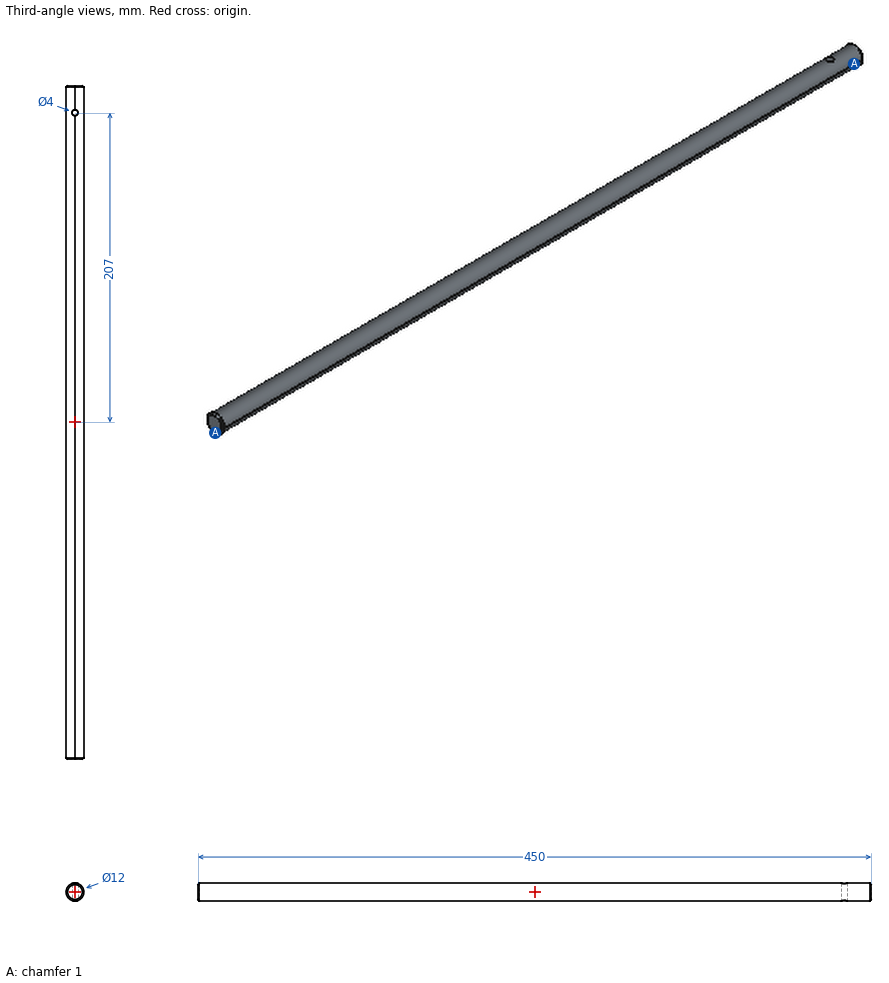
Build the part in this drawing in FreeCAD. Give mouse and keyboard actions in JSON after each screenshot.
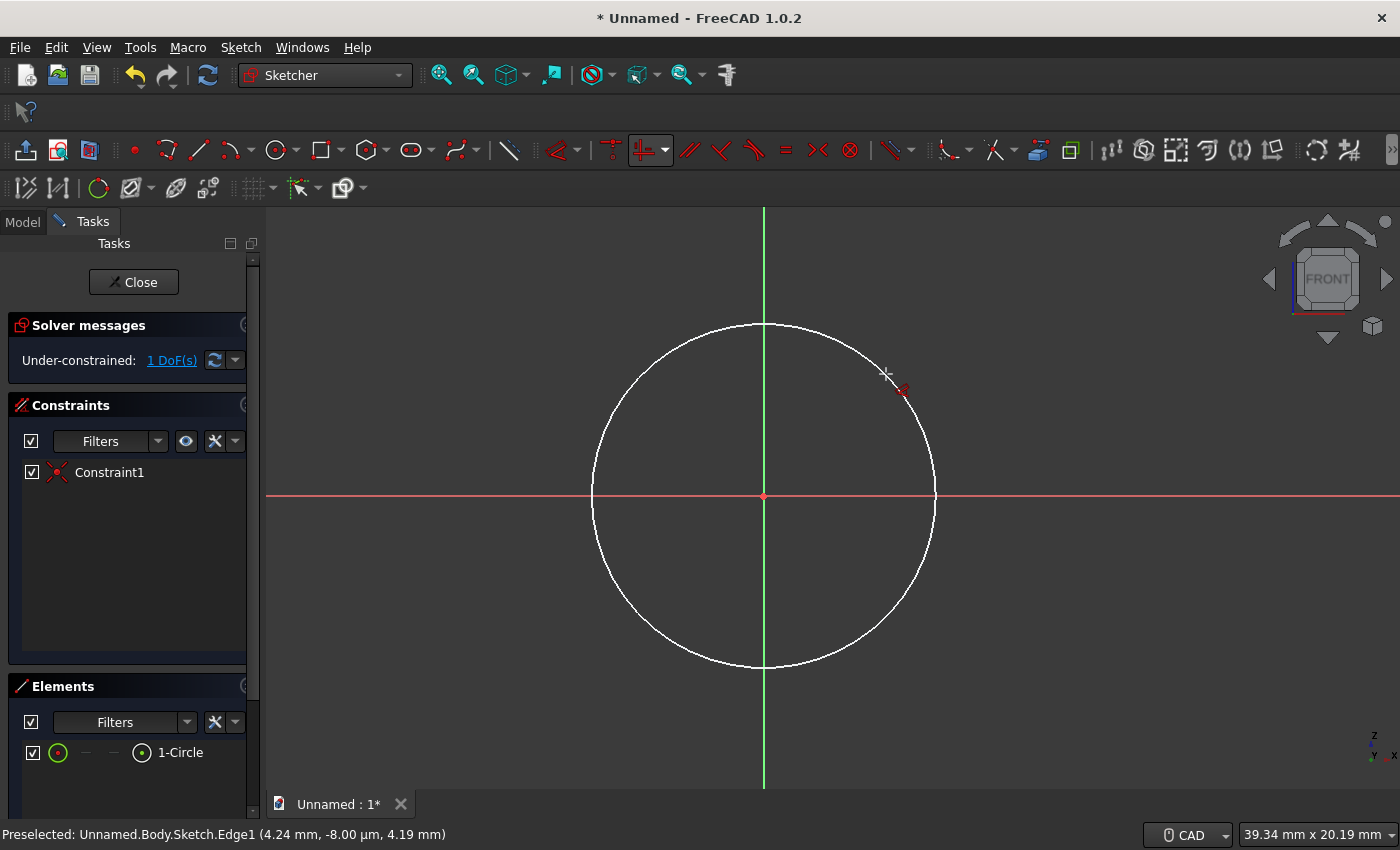
{"action": "left_click", "coordinate": [885, 374]}
{"action": "left_click", "coordinate": [908, 351]}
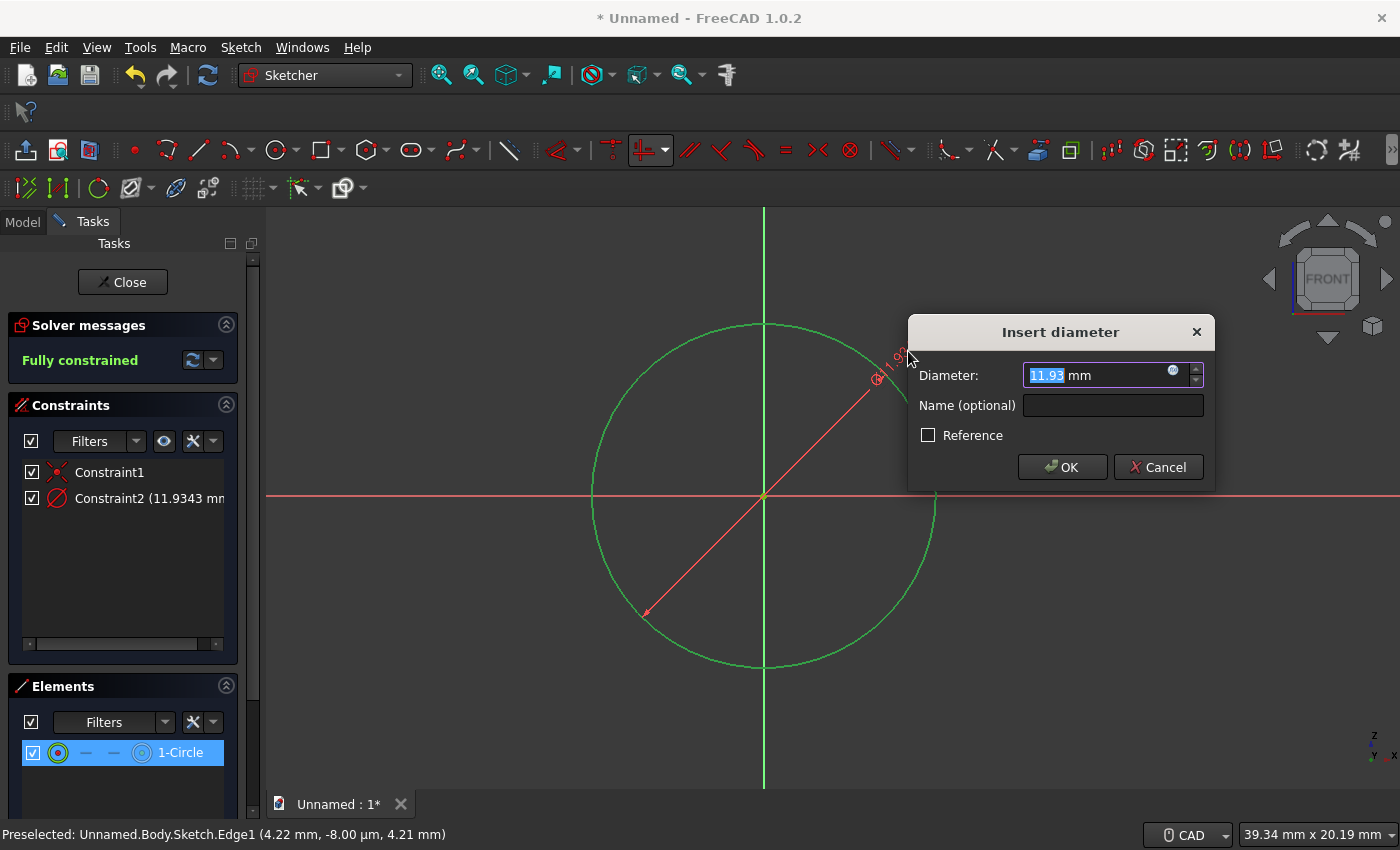
{"action": "type", "text": "12"}
{"action": "key", "text": "Return"}
{"action": "key", "text": "Escape"}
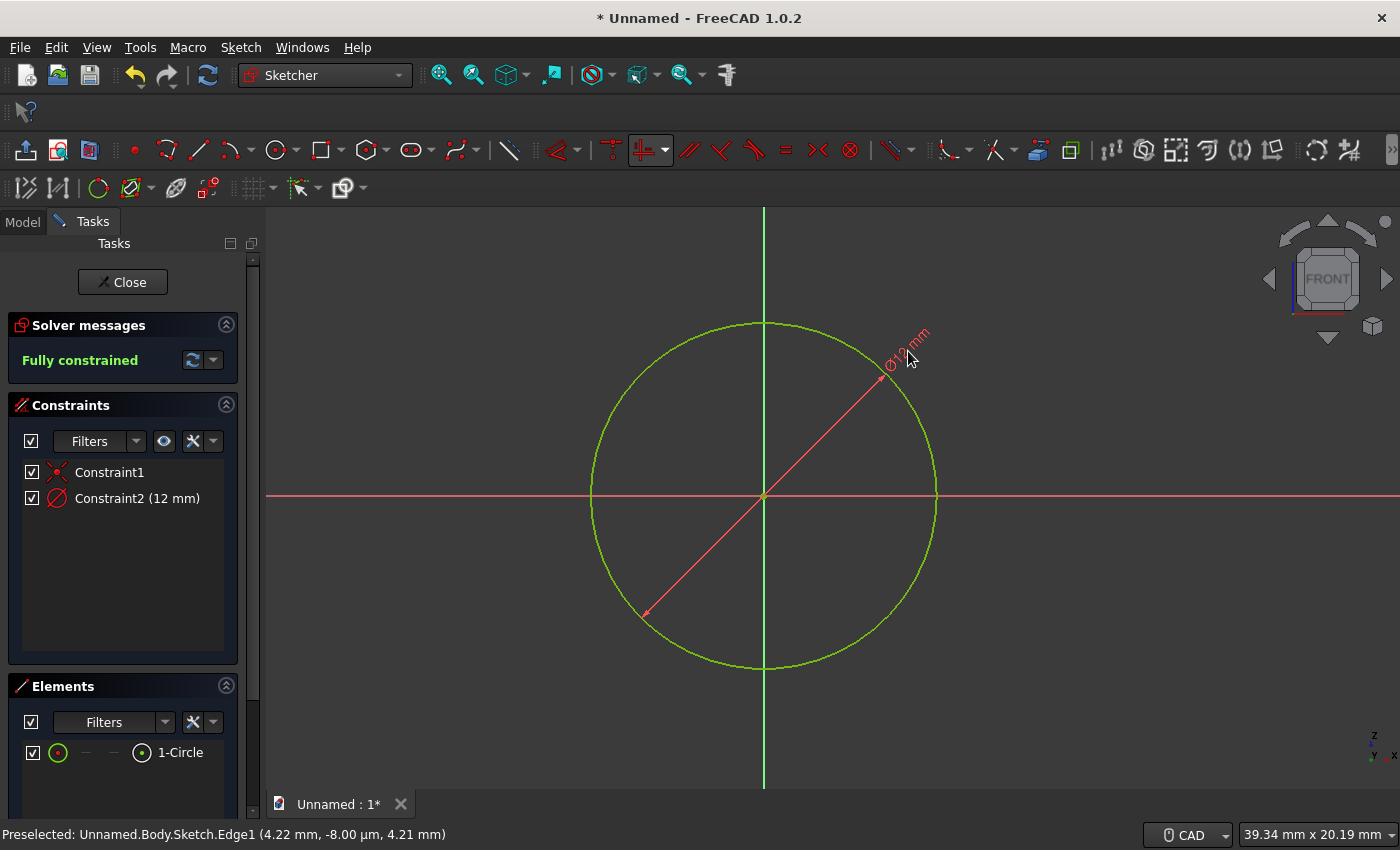
{"action": "left_click", "coordinate": [123, 282]}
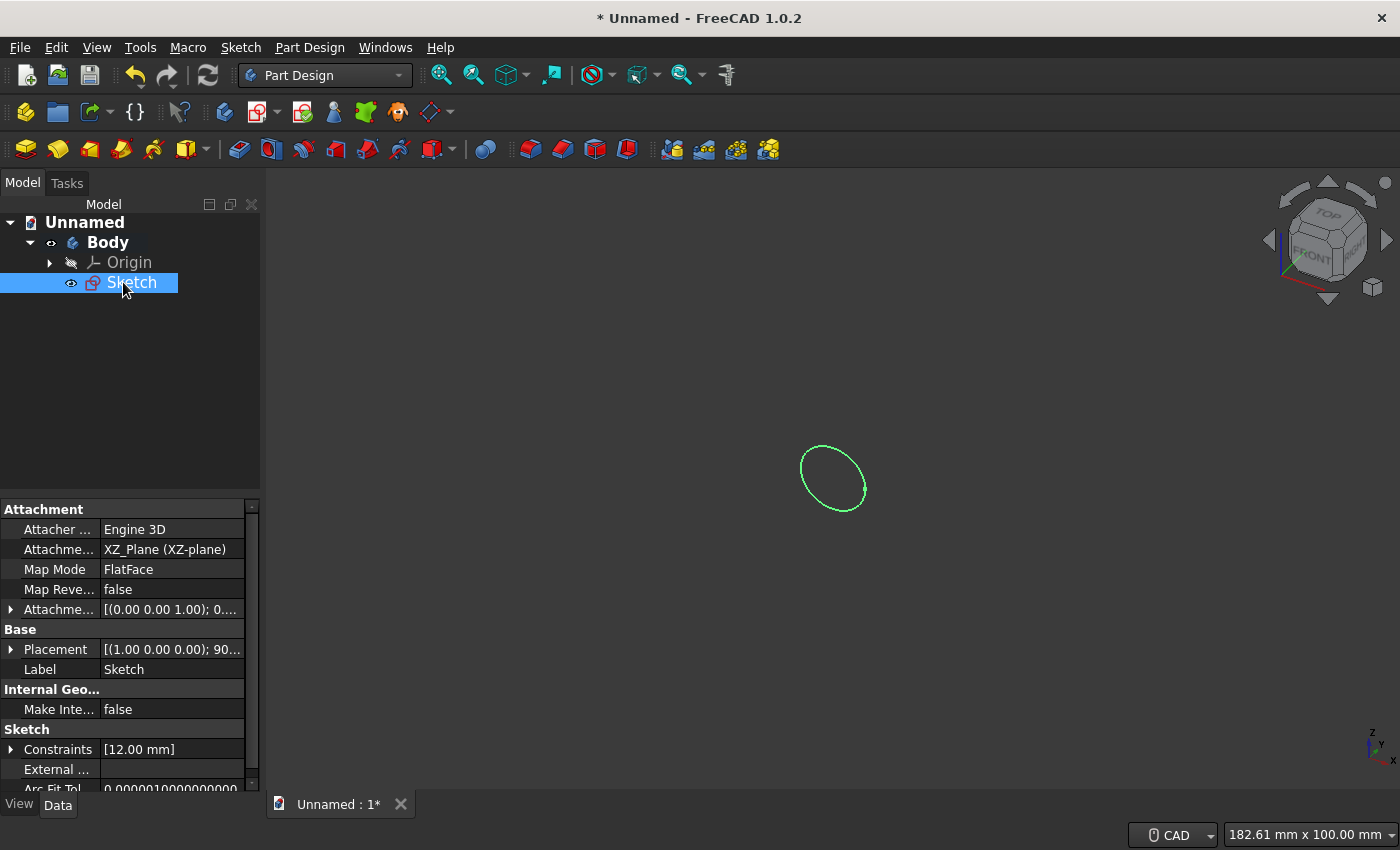
{"action": "left_click", "coordinate": [26, 150]}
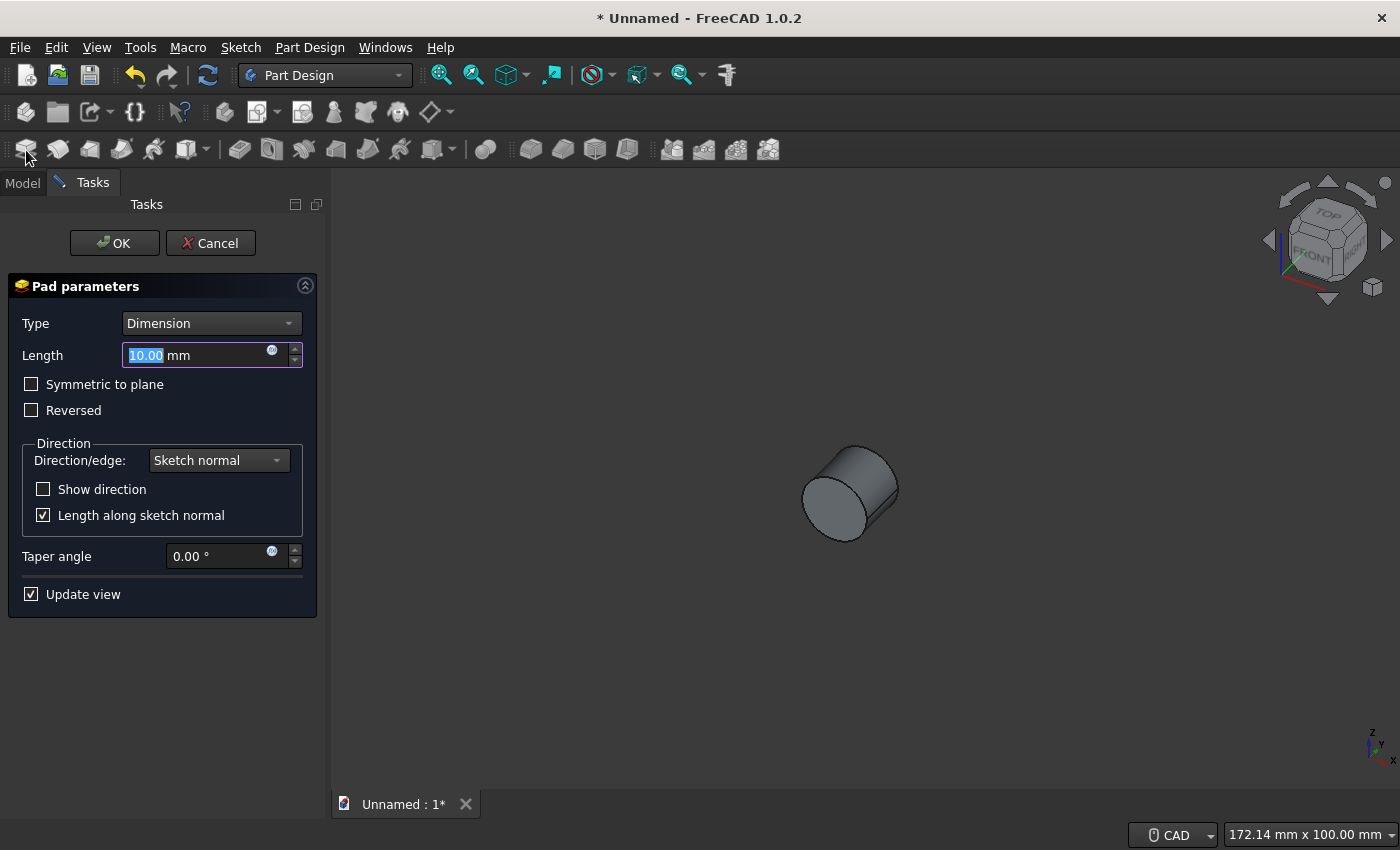
{"action": "type", "text": "450"}
{"action": "key", "text": "Tab"}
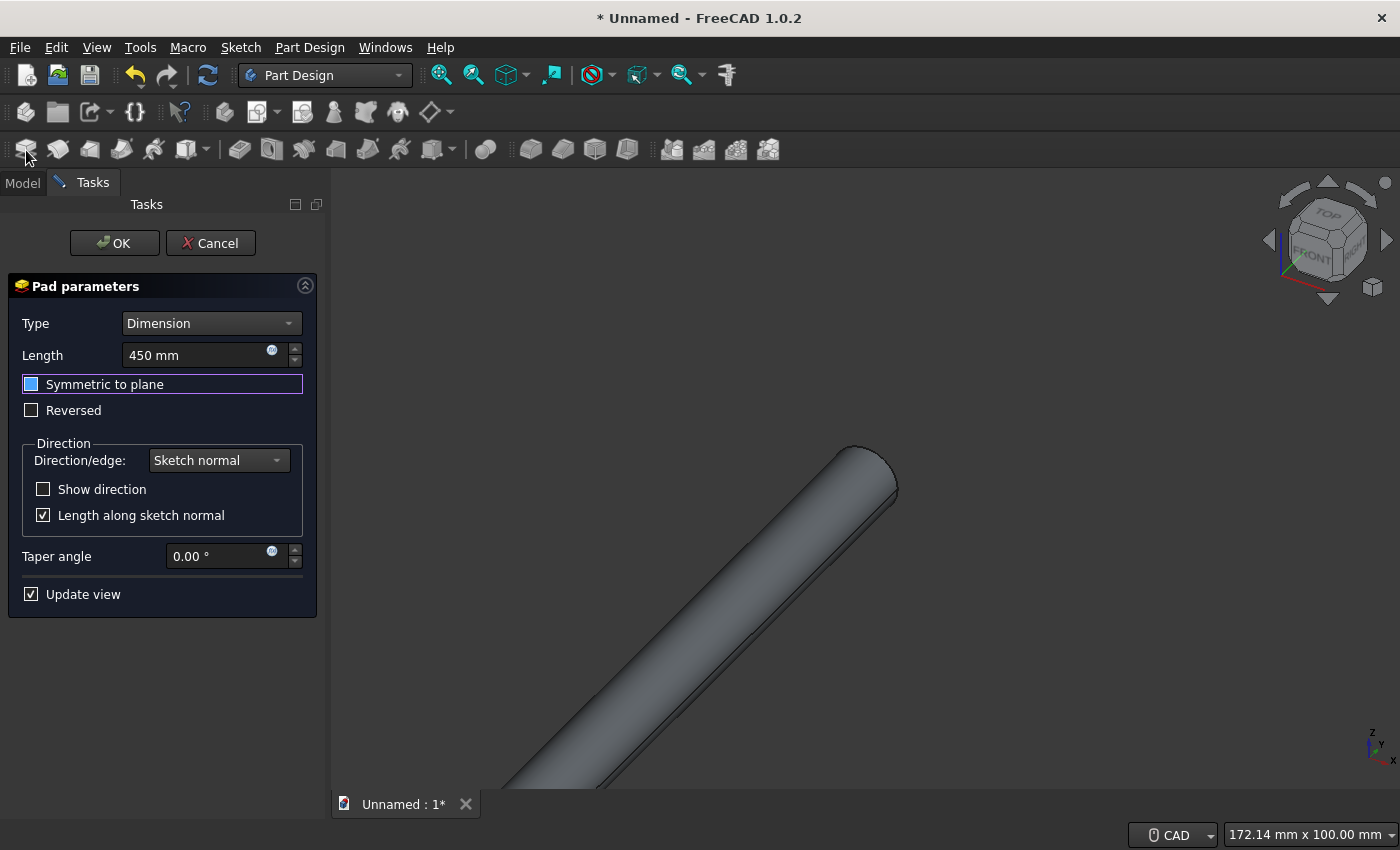
{"action": "left_click", "coordinate": [30, 384]}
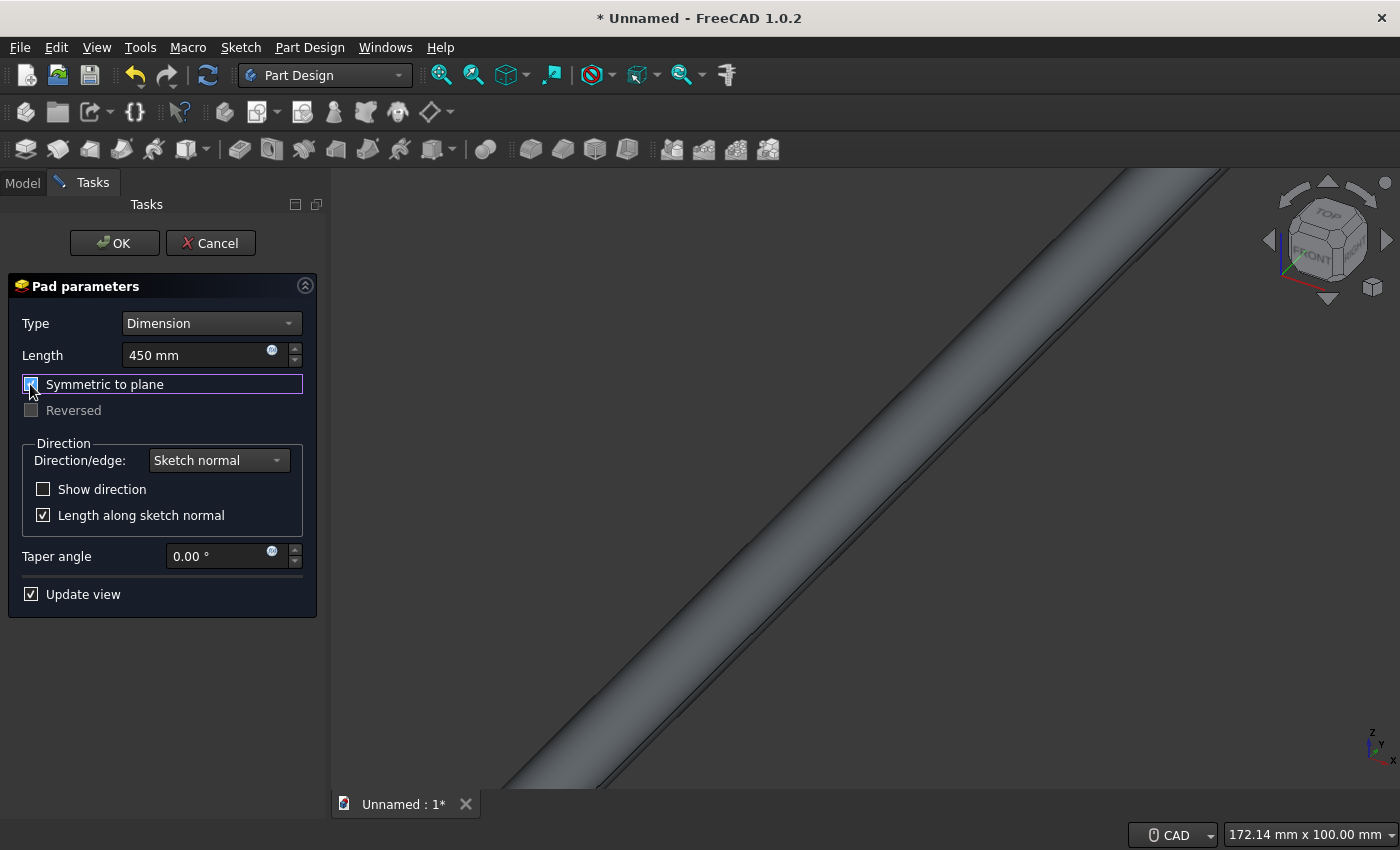
{"action": "left_click", "coordinate": [115, 243]}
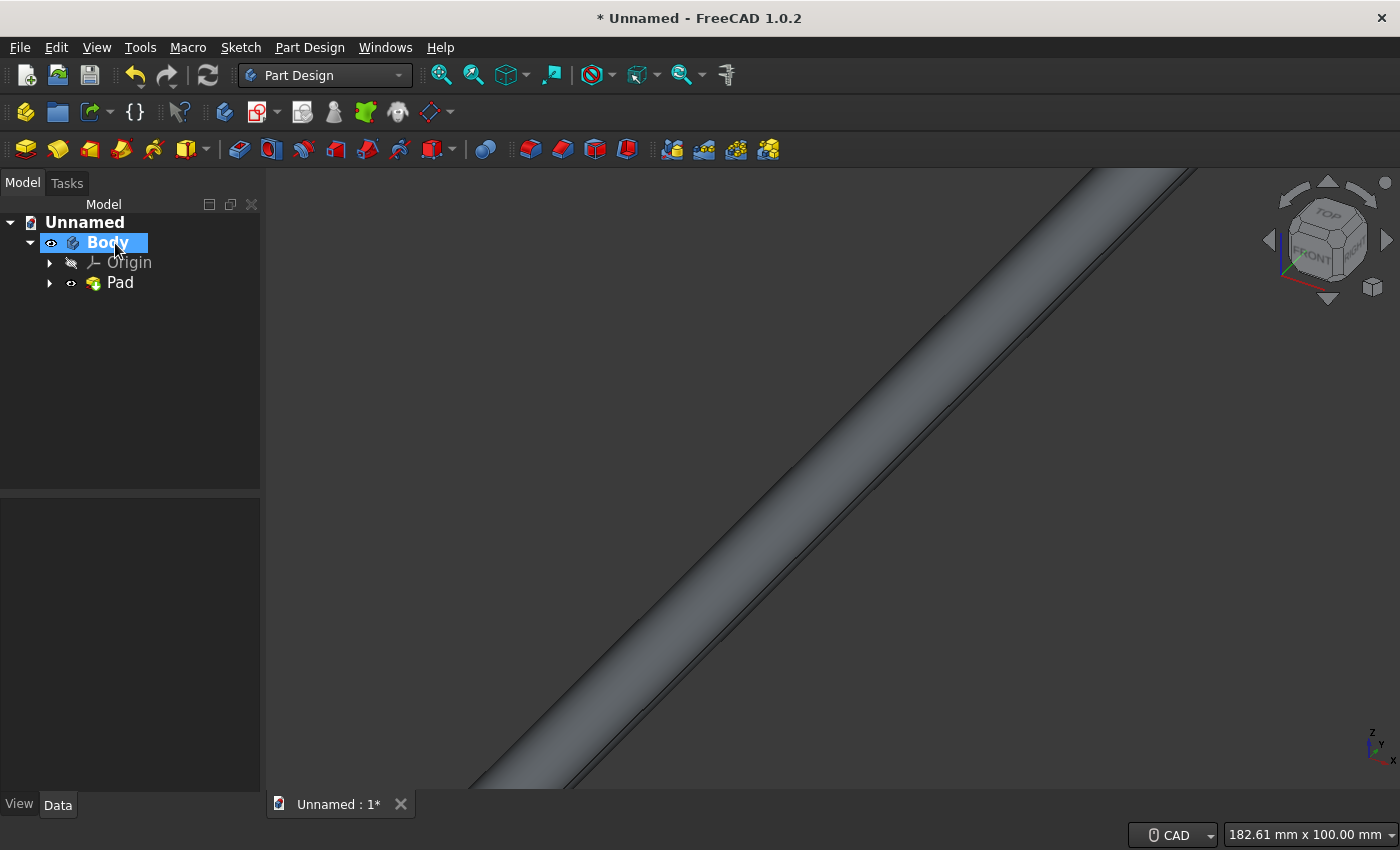
{"action": "key", "text": "v f"}